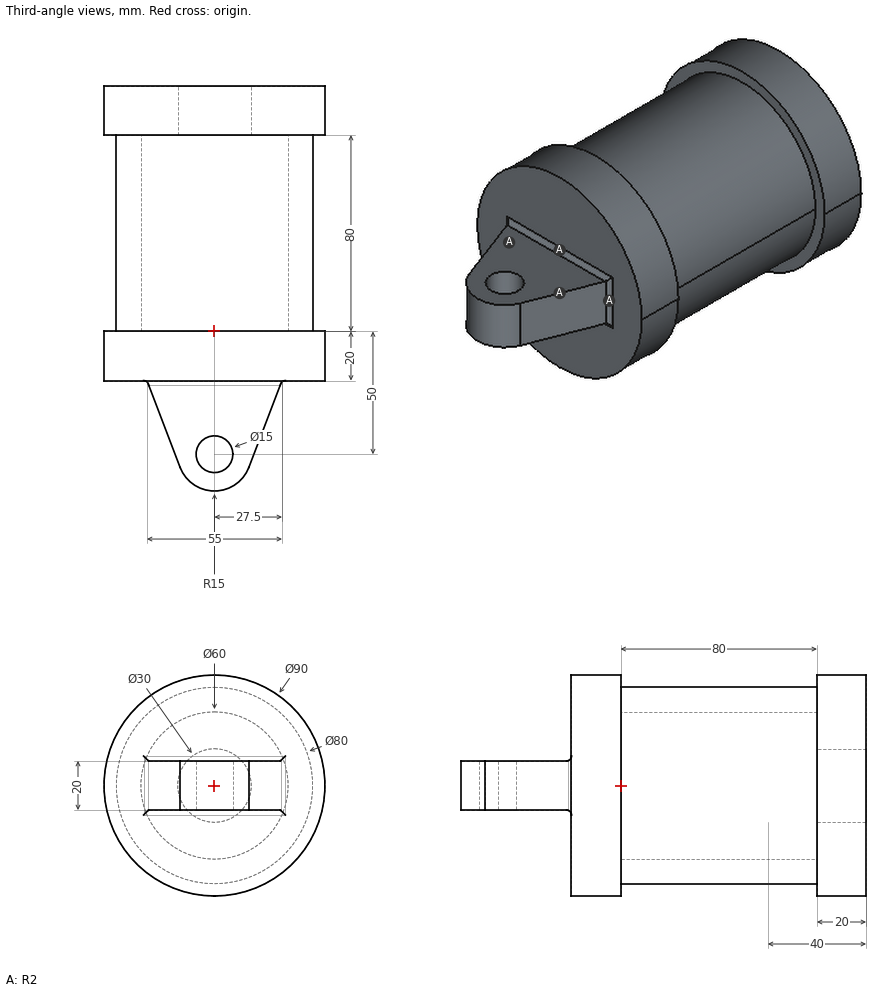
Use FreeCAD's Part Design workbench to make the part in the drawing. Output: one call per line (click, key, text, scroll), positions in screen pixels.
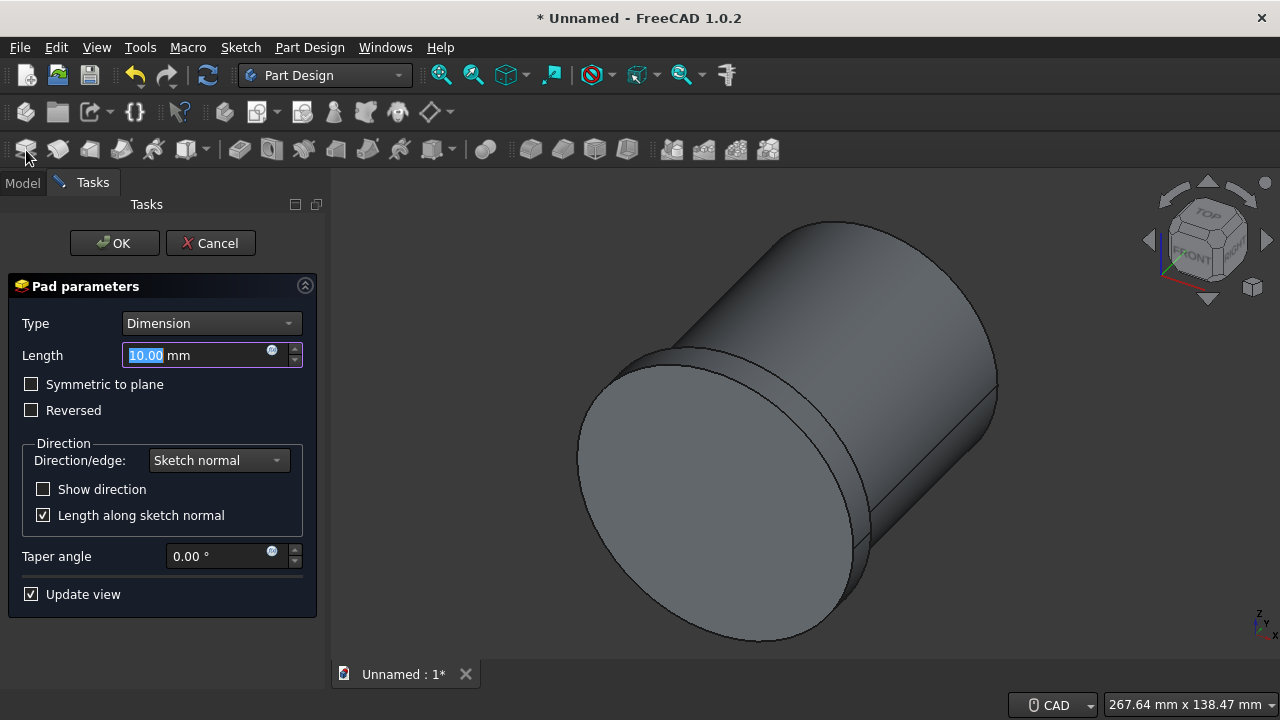
text(20)
key(Tab)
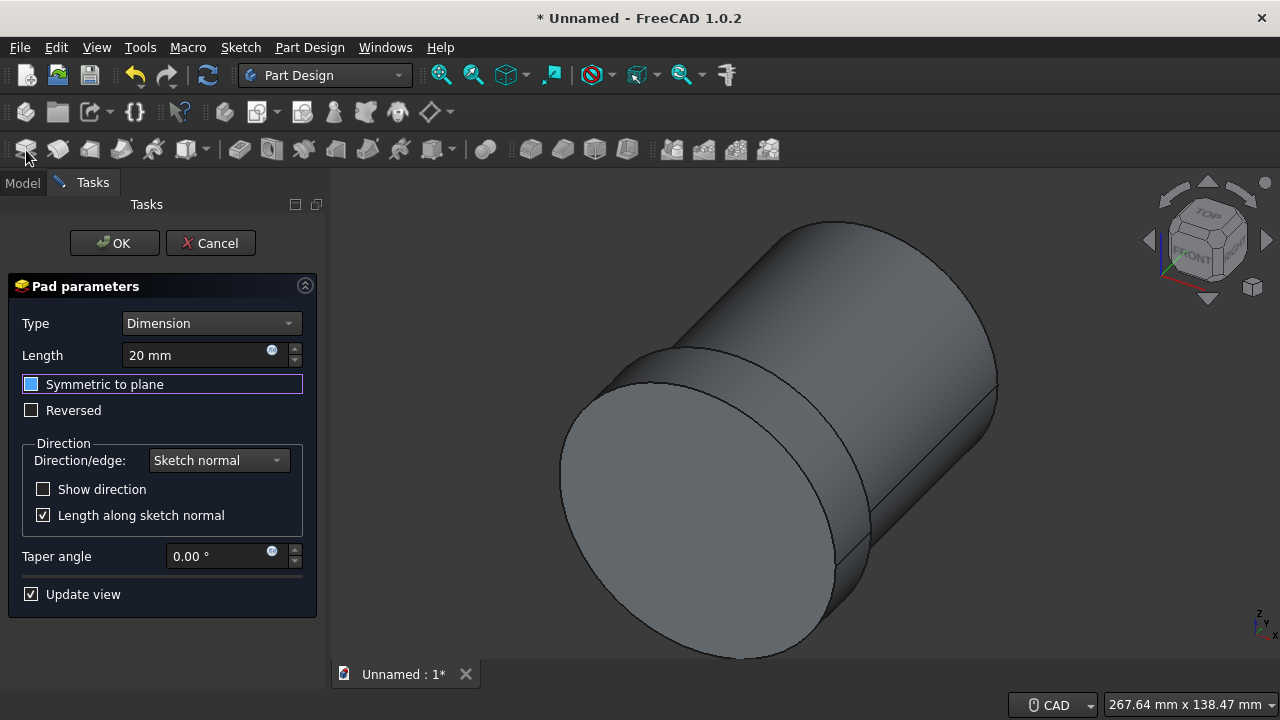
click(115, 243)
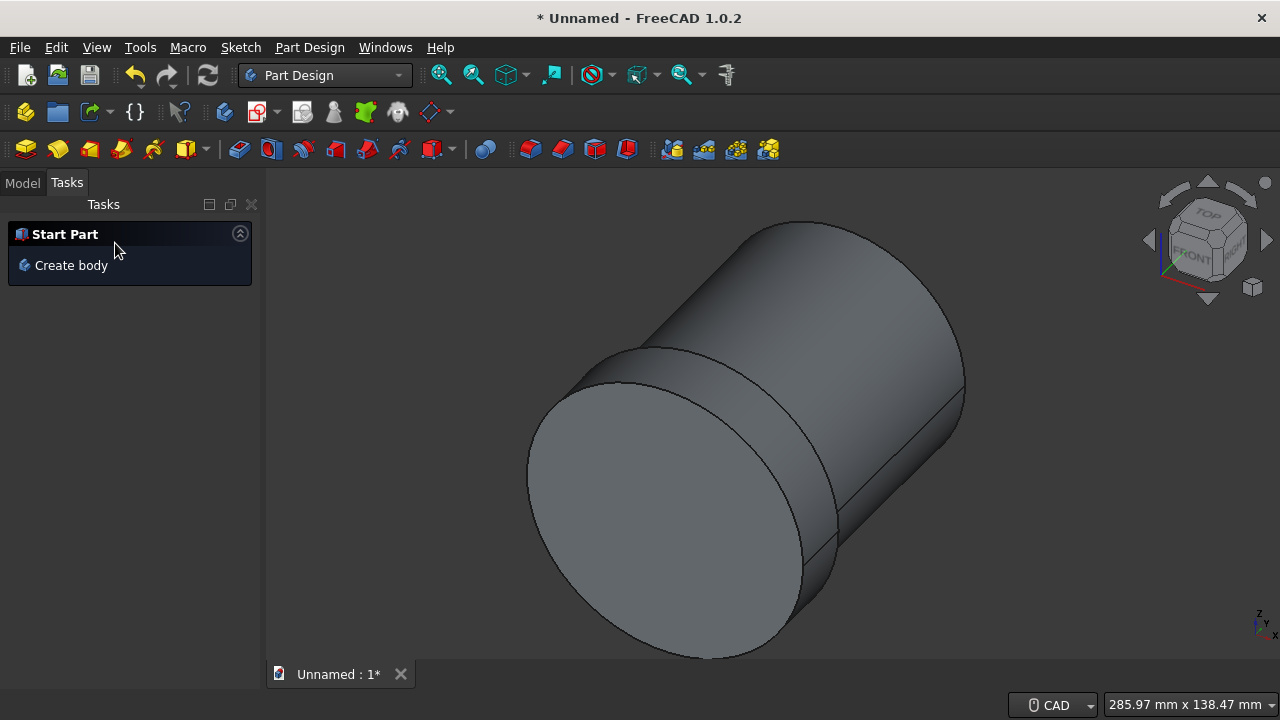
key(v)
key(f)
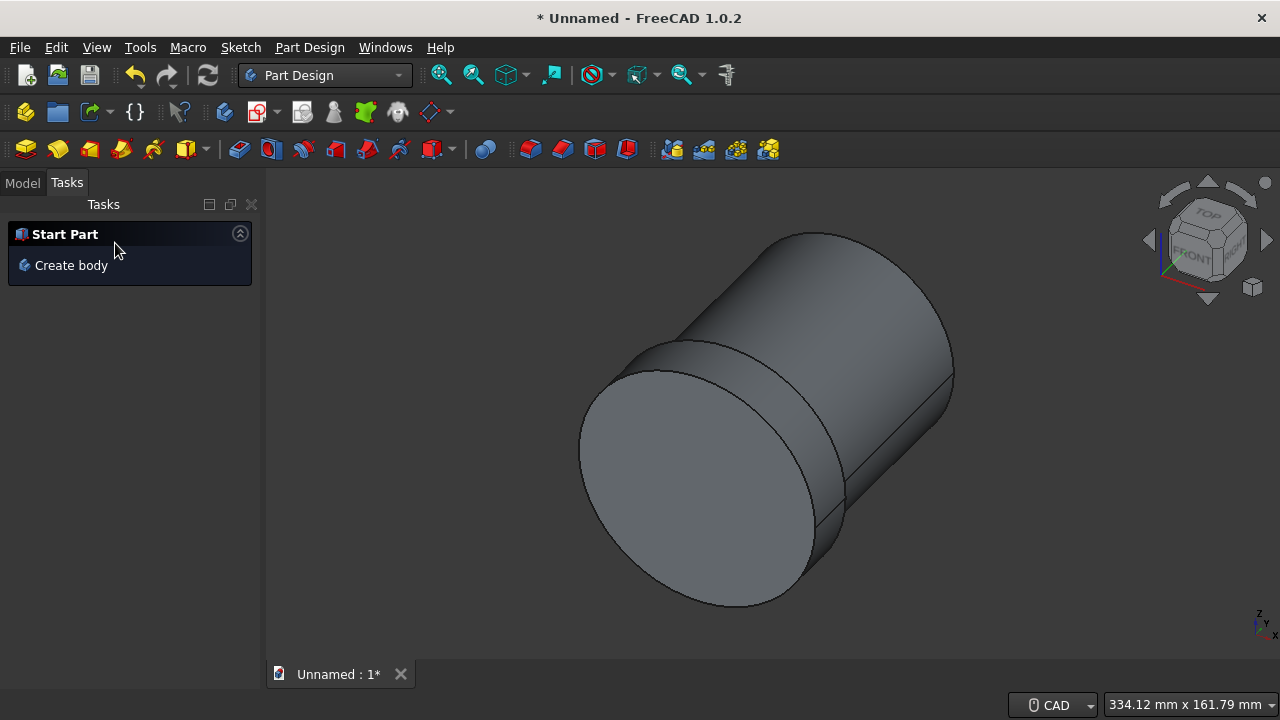
click(23, 182)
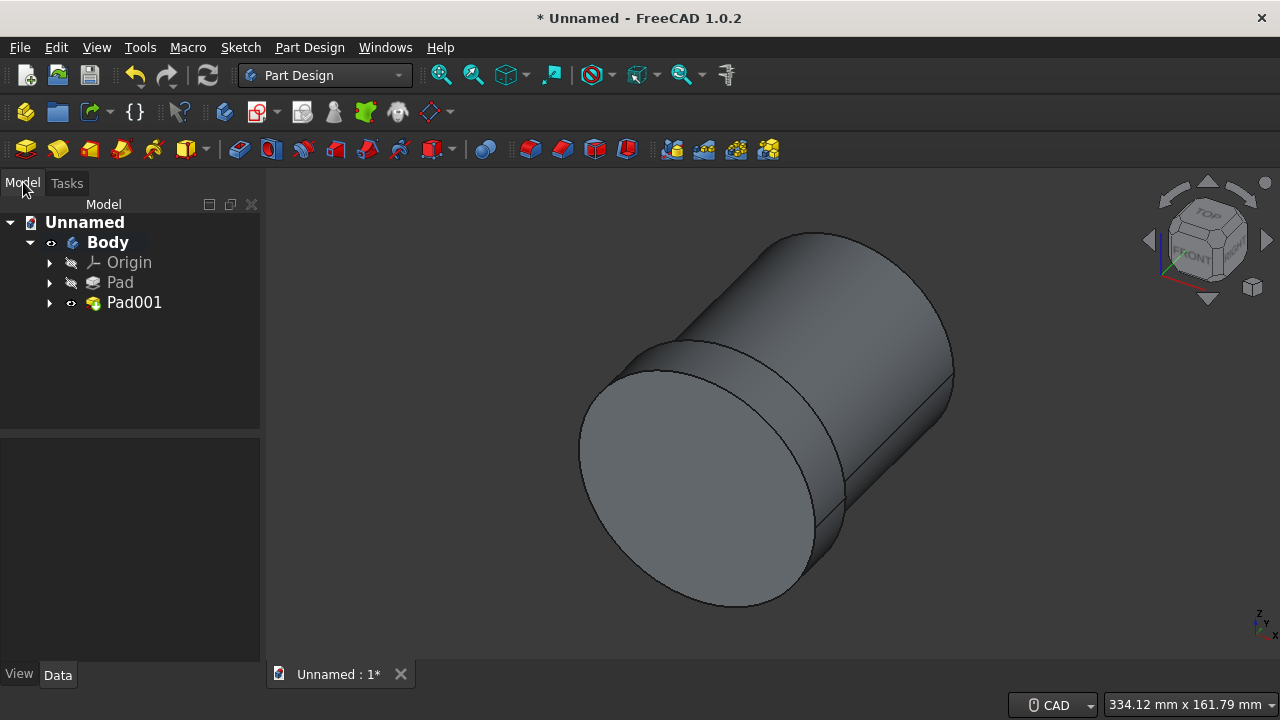
click(50, 263)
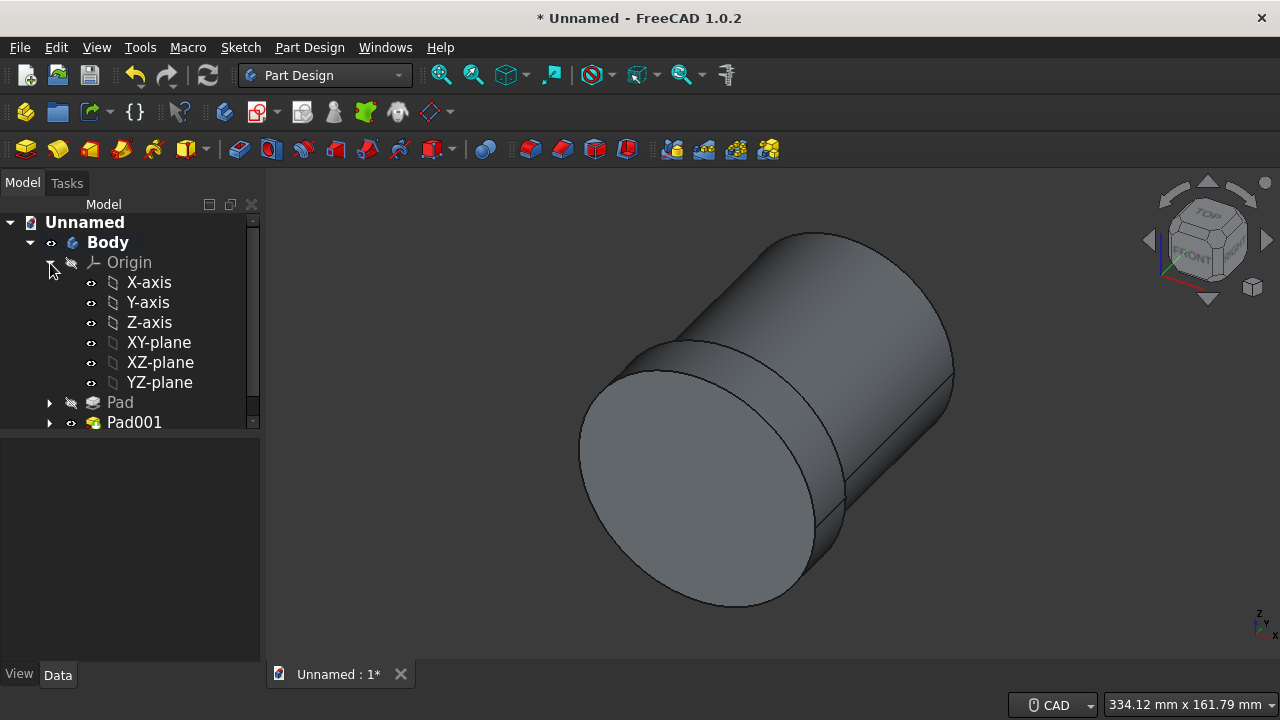
click(136, 363)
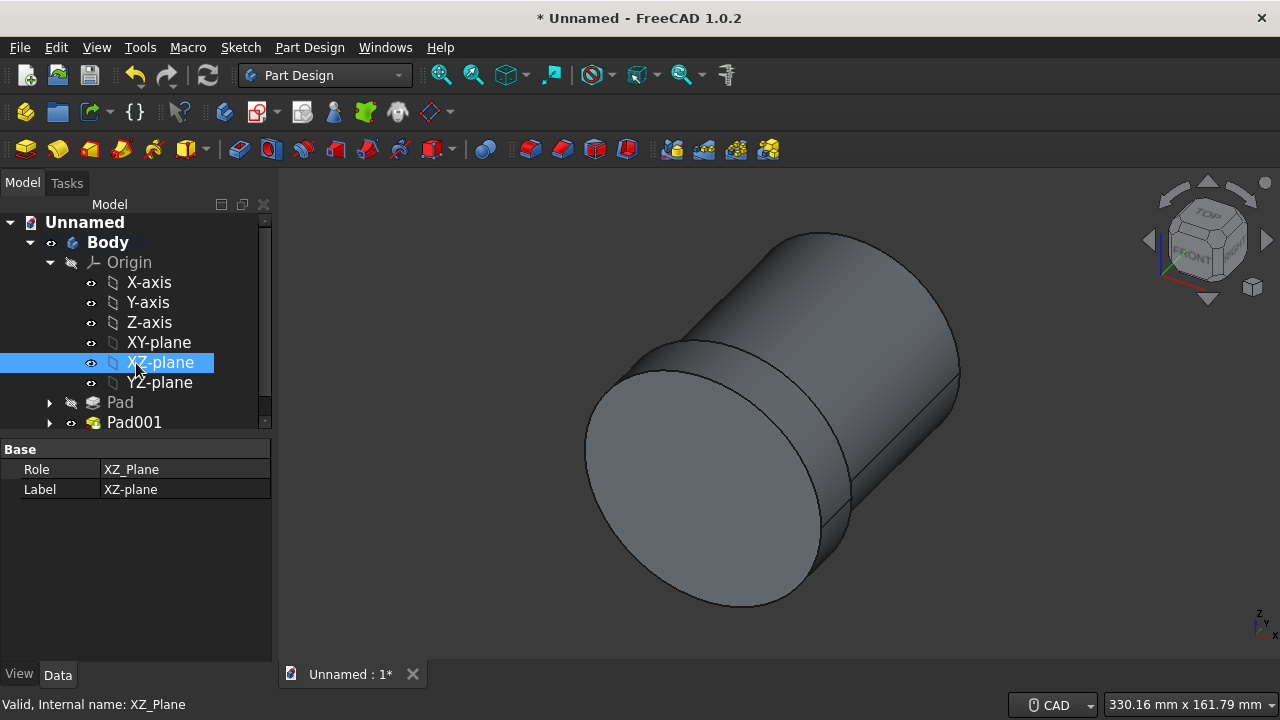
click(430, 112)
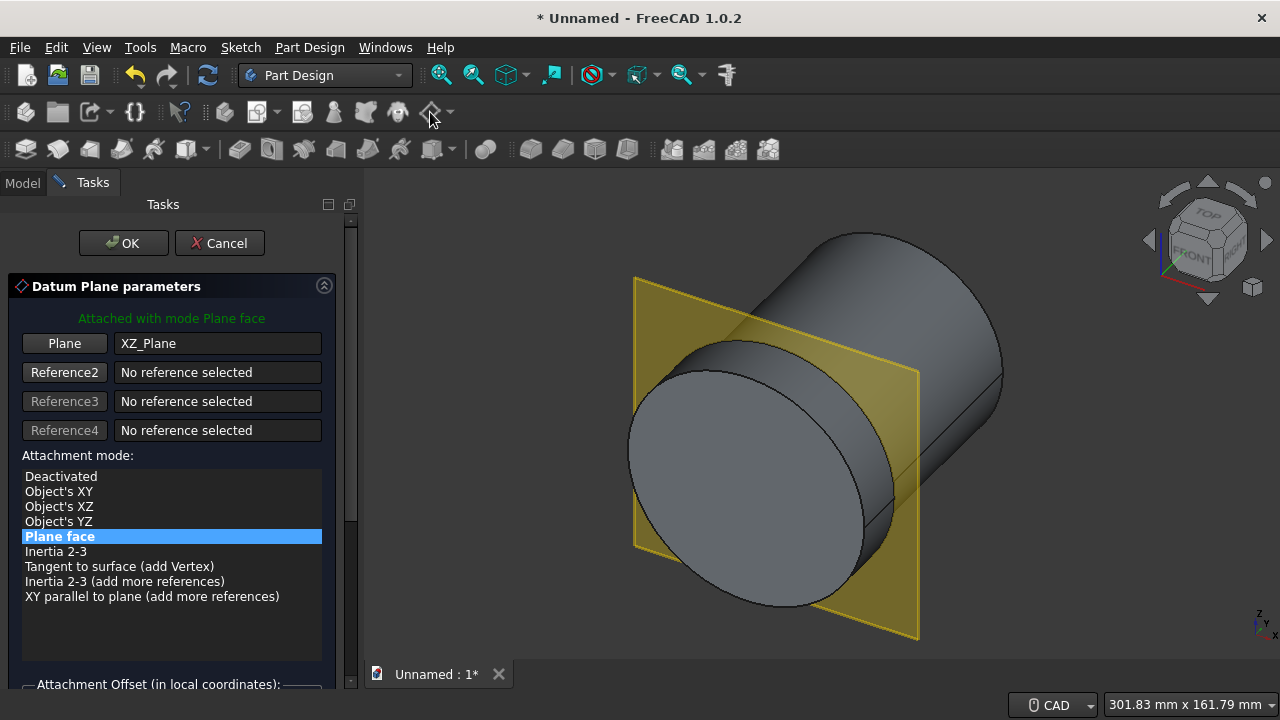
scroll(351, 451, down, 3)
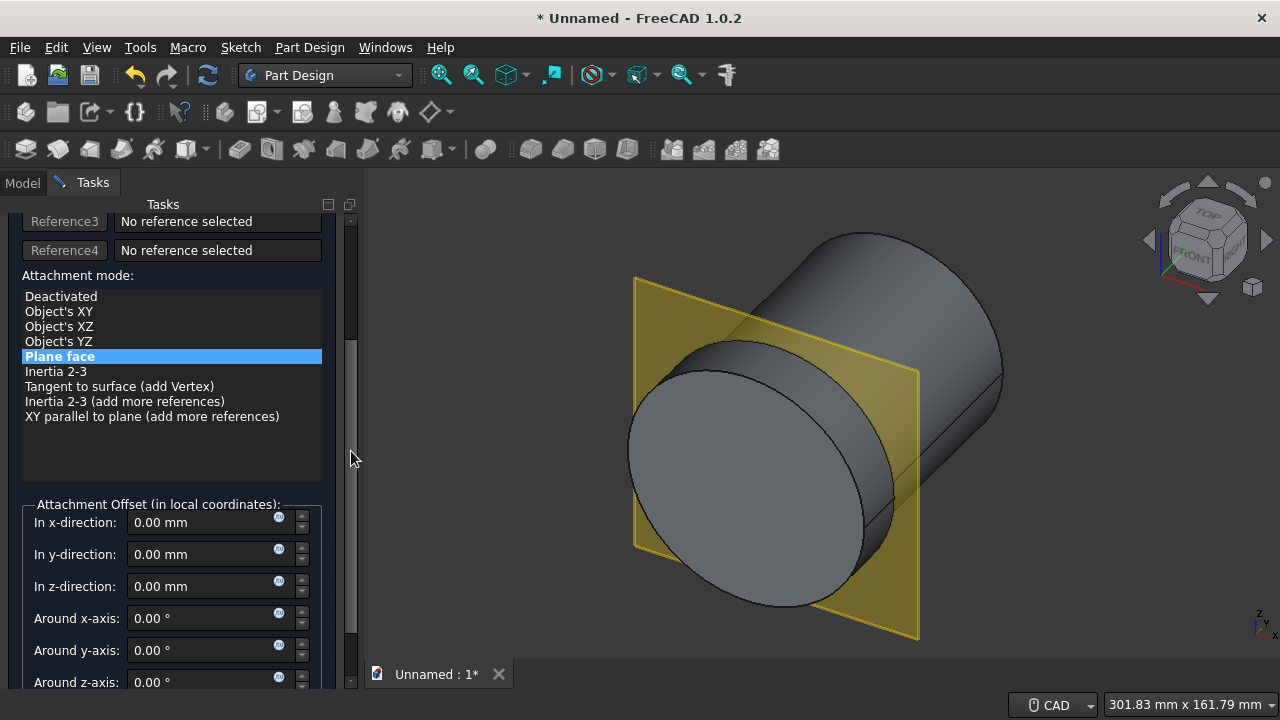
triple_click(210, 586)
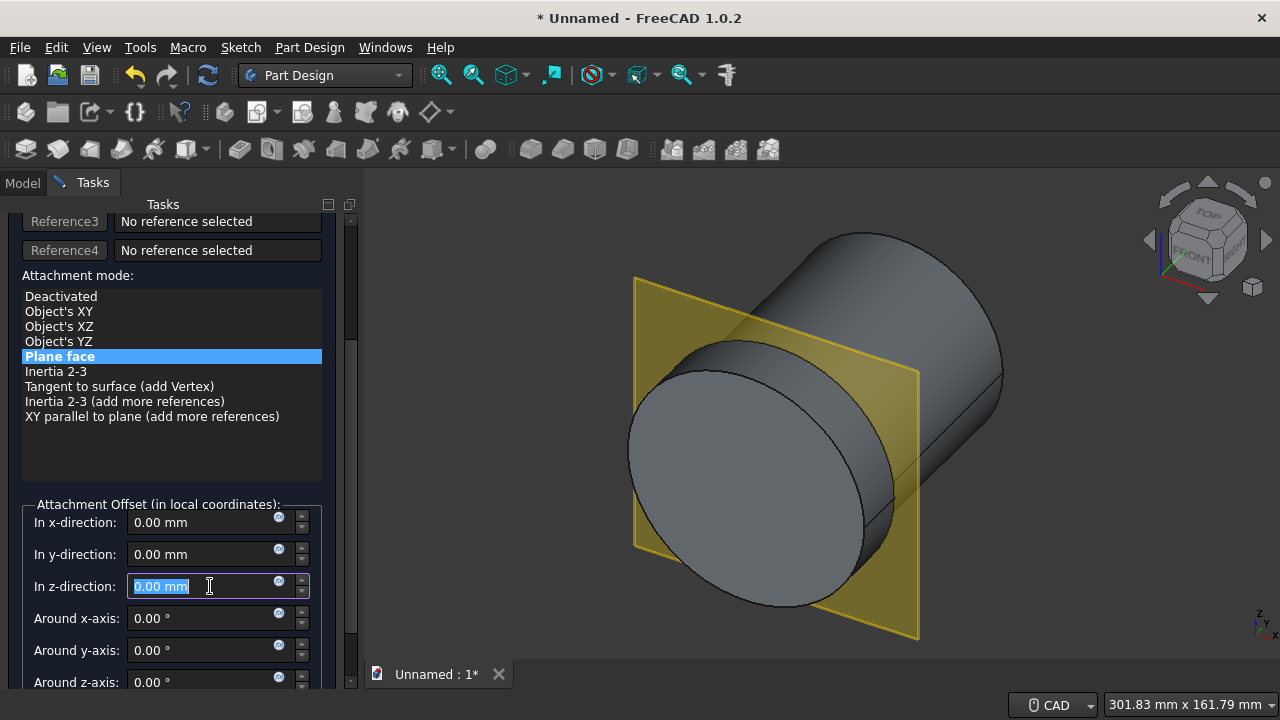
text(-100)
key(Tab)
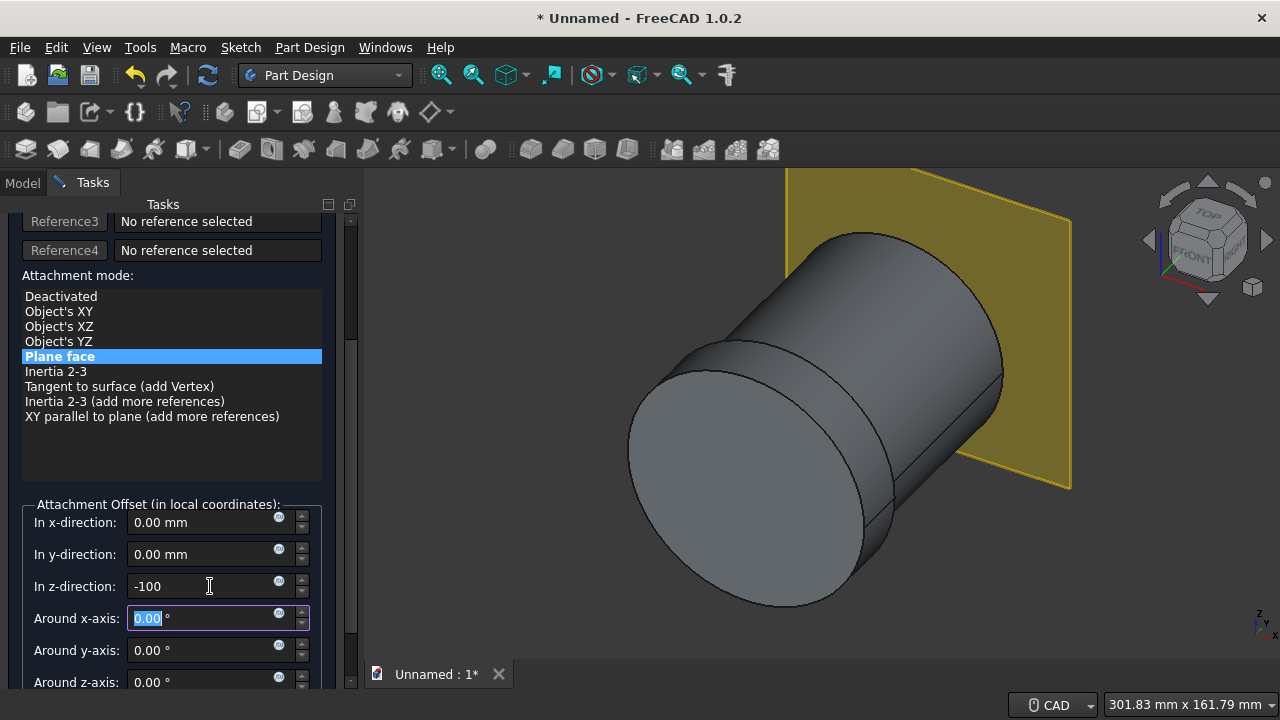
scroll(351, 451, up, 4)